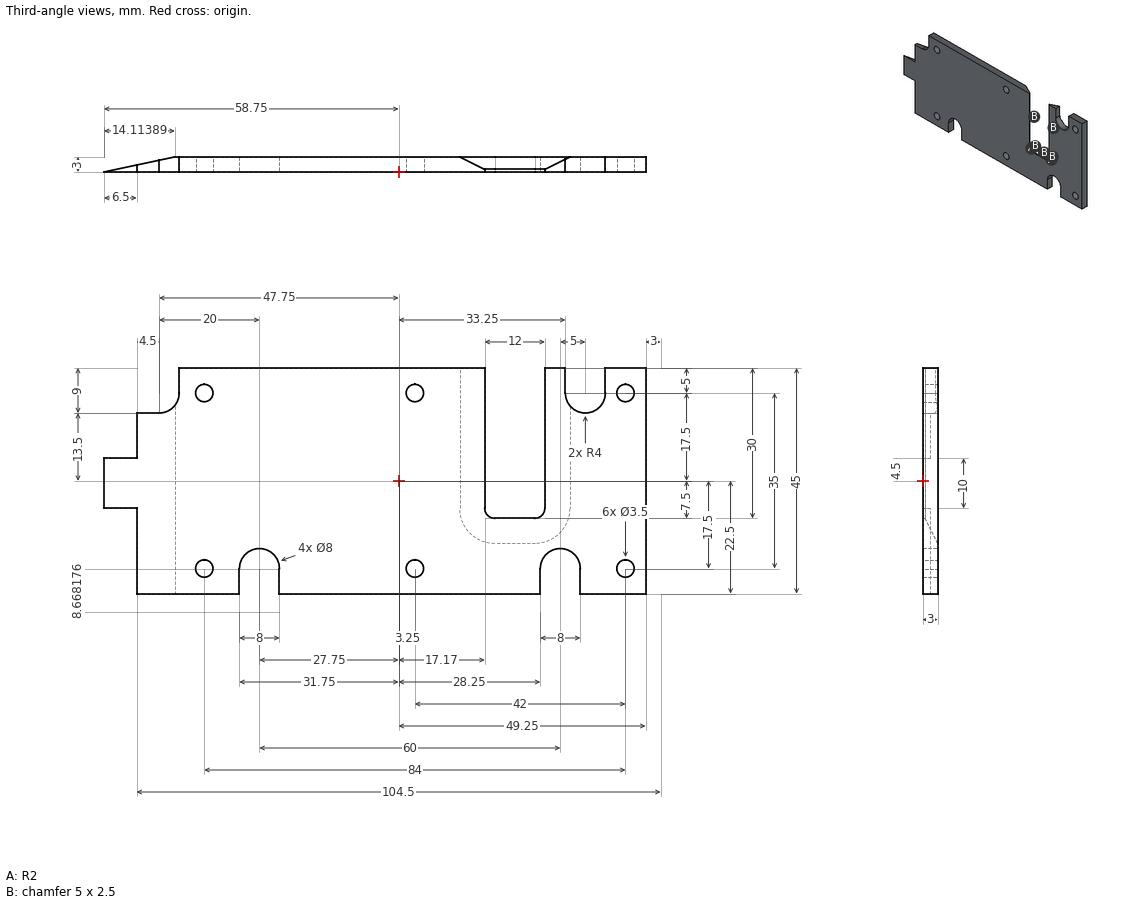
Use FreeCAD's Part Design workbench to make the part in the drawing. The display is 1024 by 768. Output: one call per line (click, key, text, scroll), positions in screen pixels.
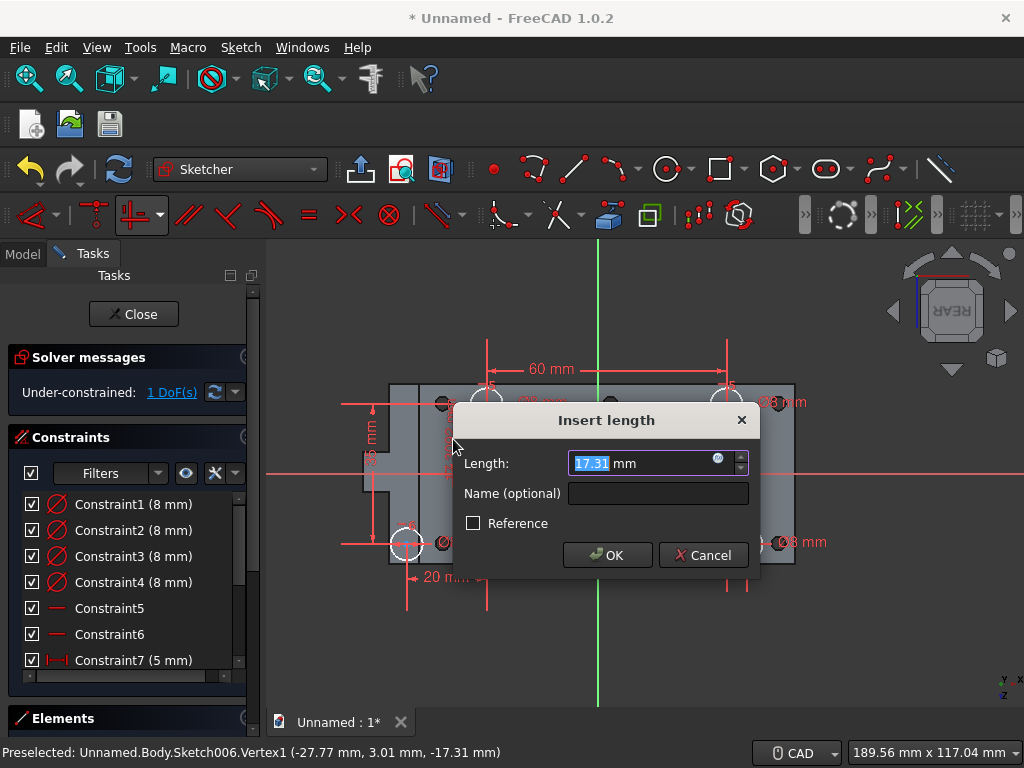
text(17.5)
key(Return)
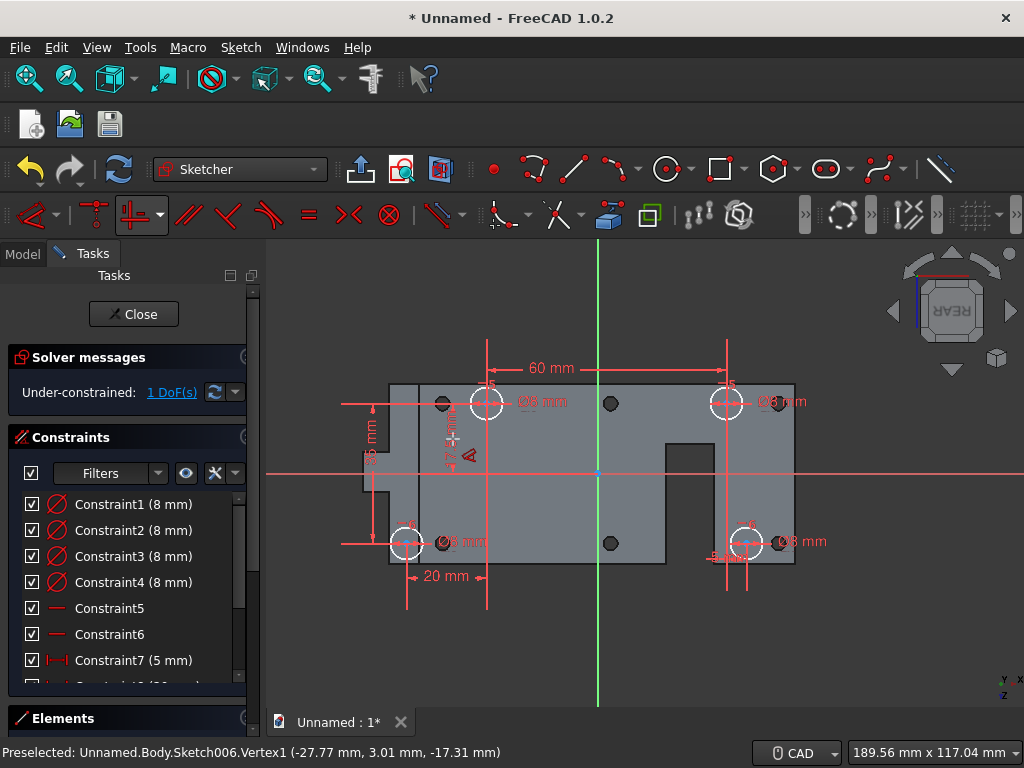
click(487, 404)
click(542, 508)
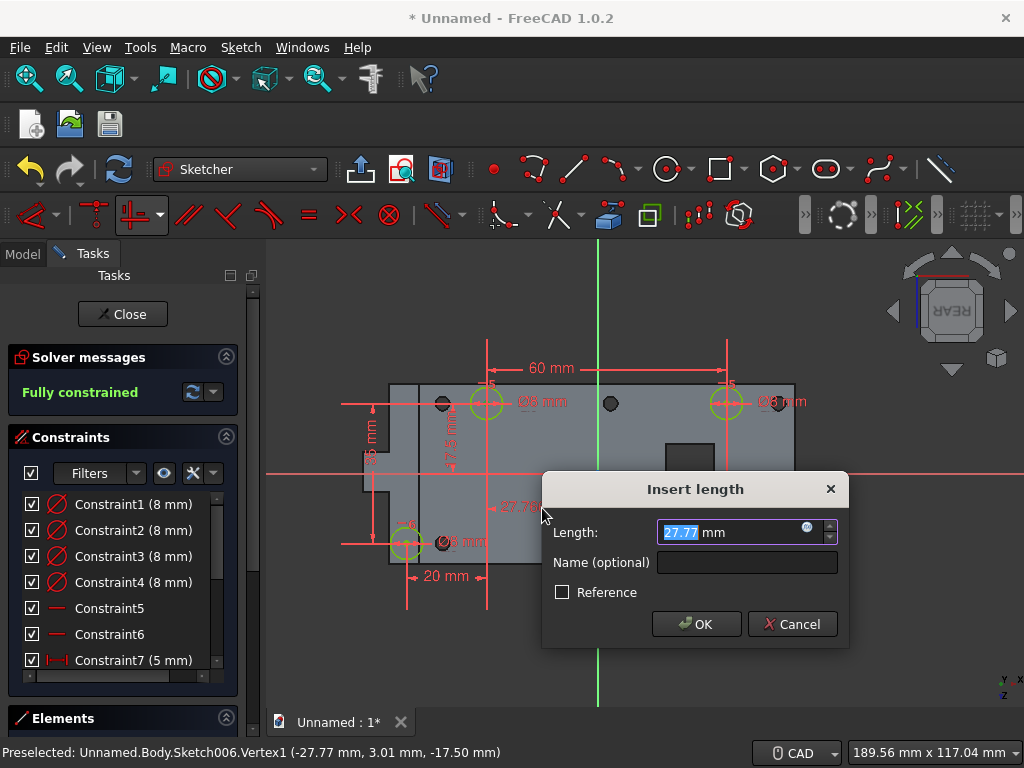
text(27.75)
key(Return)
key(Escape)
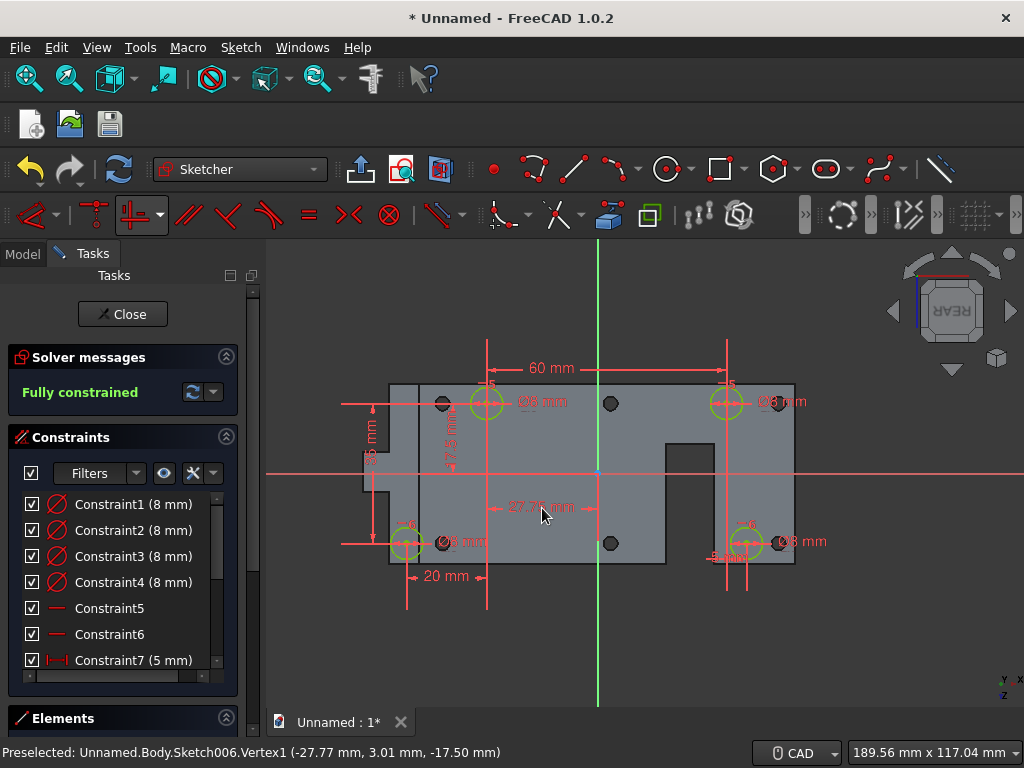
click(123, 314)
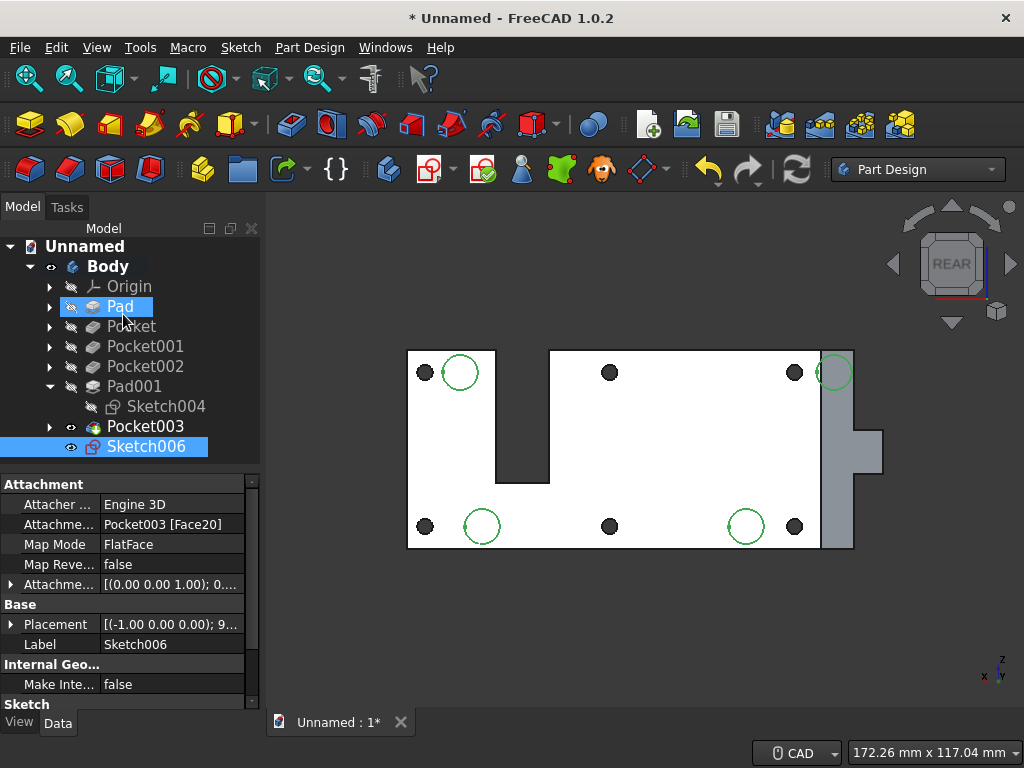
click(292, 124)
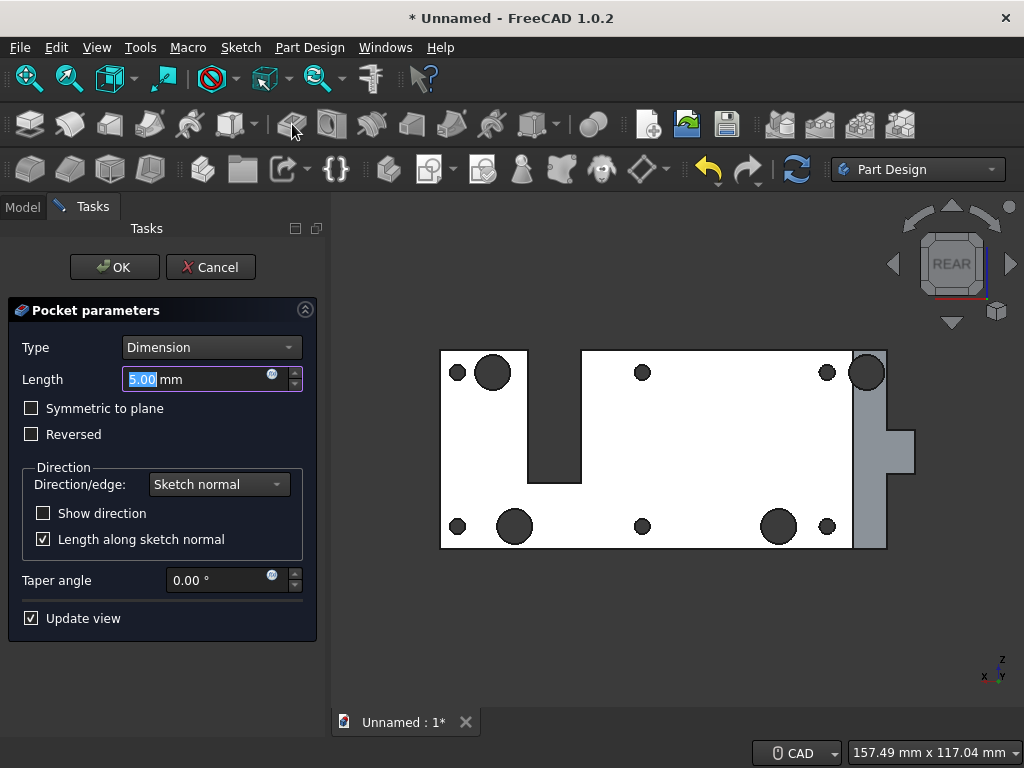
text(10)
key(Tab)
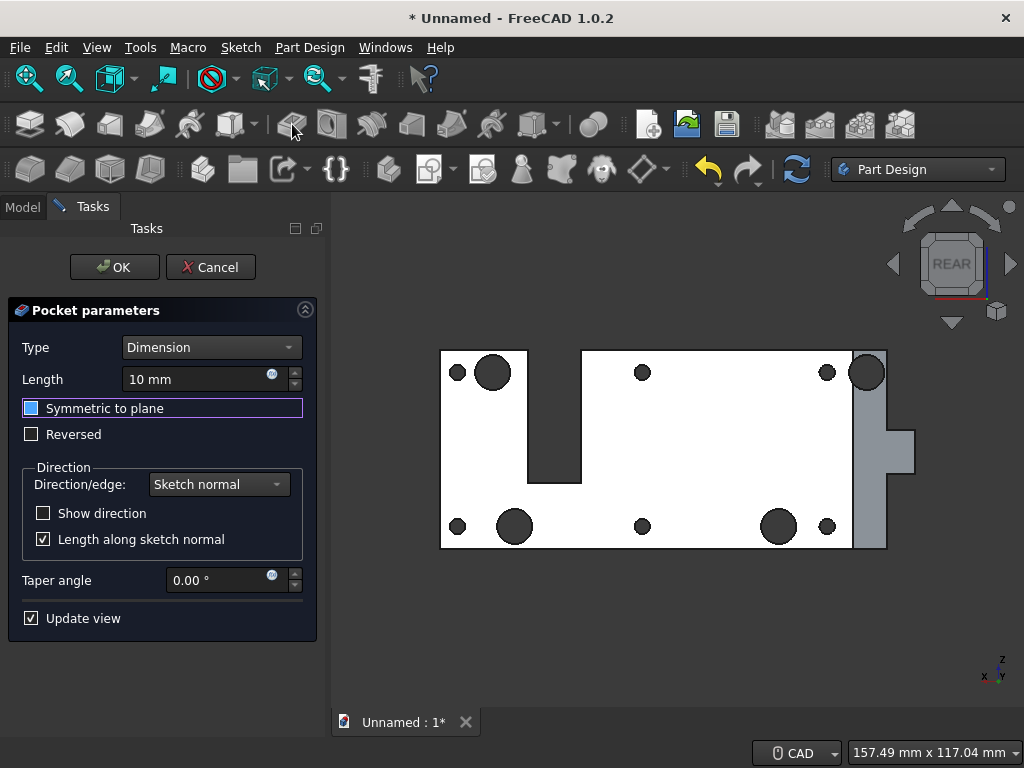
click(115, 267)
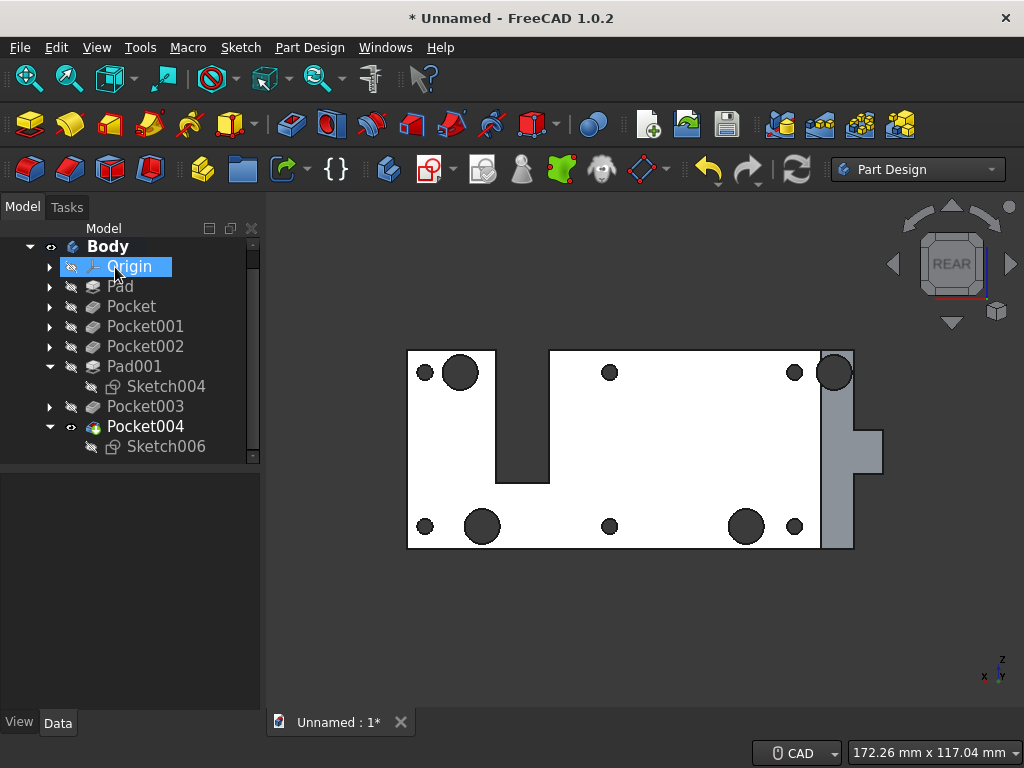
click(673, 448)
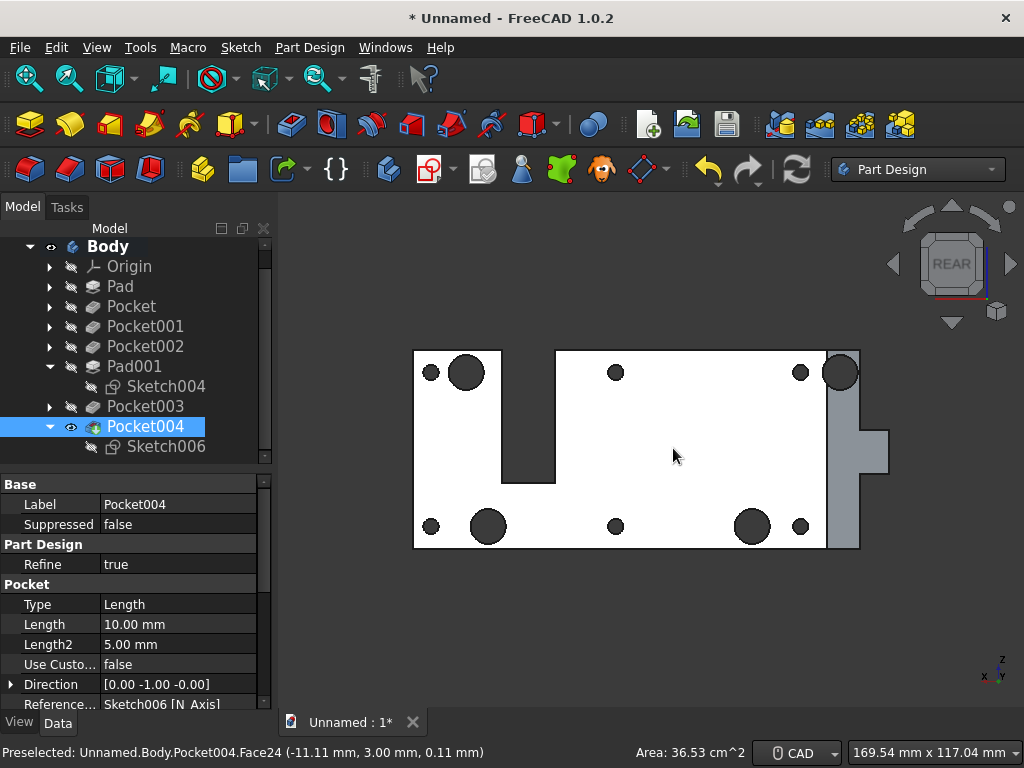
click(430, 170)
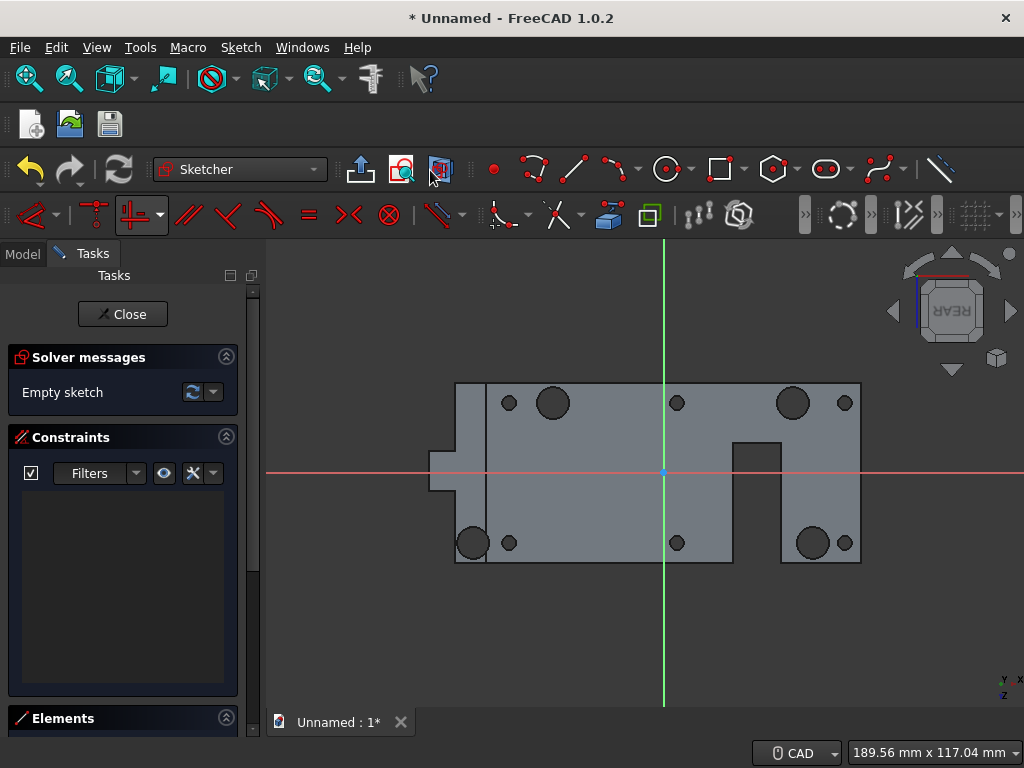
key(g)
key(r)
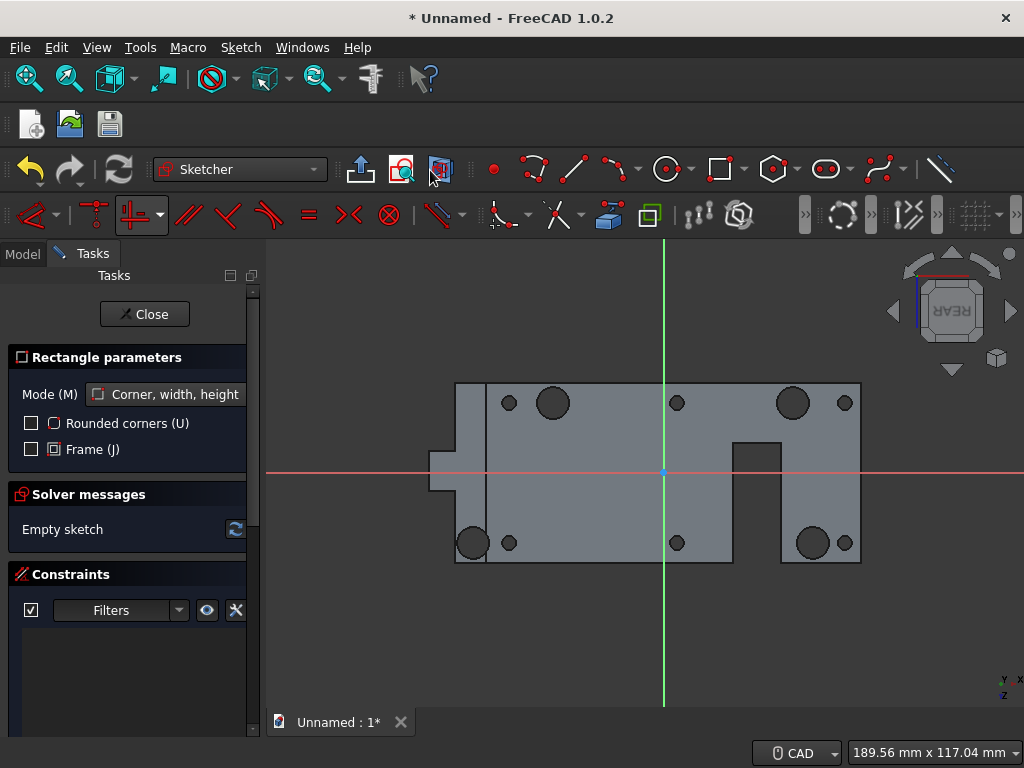
click(537, 368)
move(569, 403)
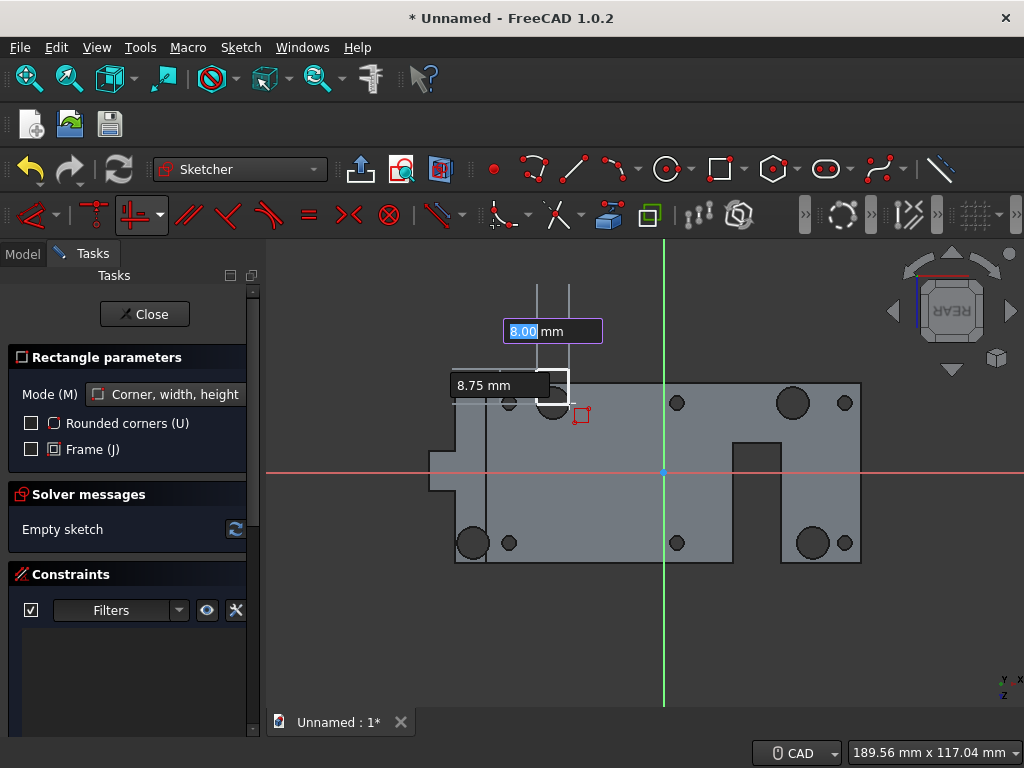
text(8)
key(Tab)
text(8.668176)
key(Return)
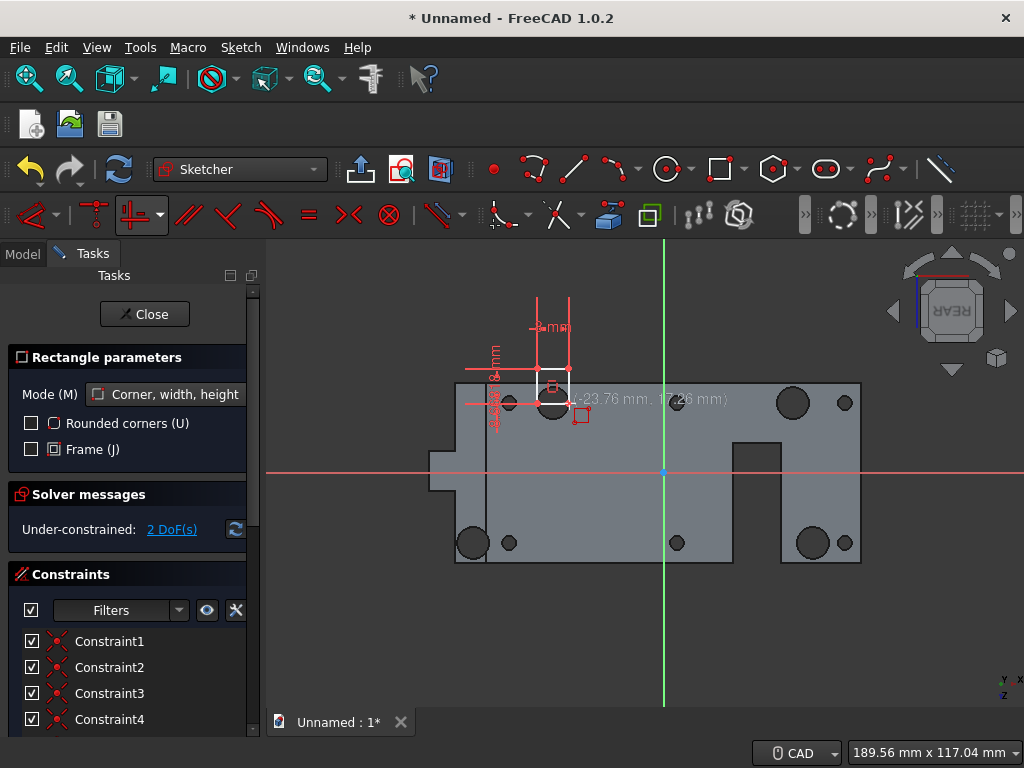
click(777, 368)
move(809, 403)